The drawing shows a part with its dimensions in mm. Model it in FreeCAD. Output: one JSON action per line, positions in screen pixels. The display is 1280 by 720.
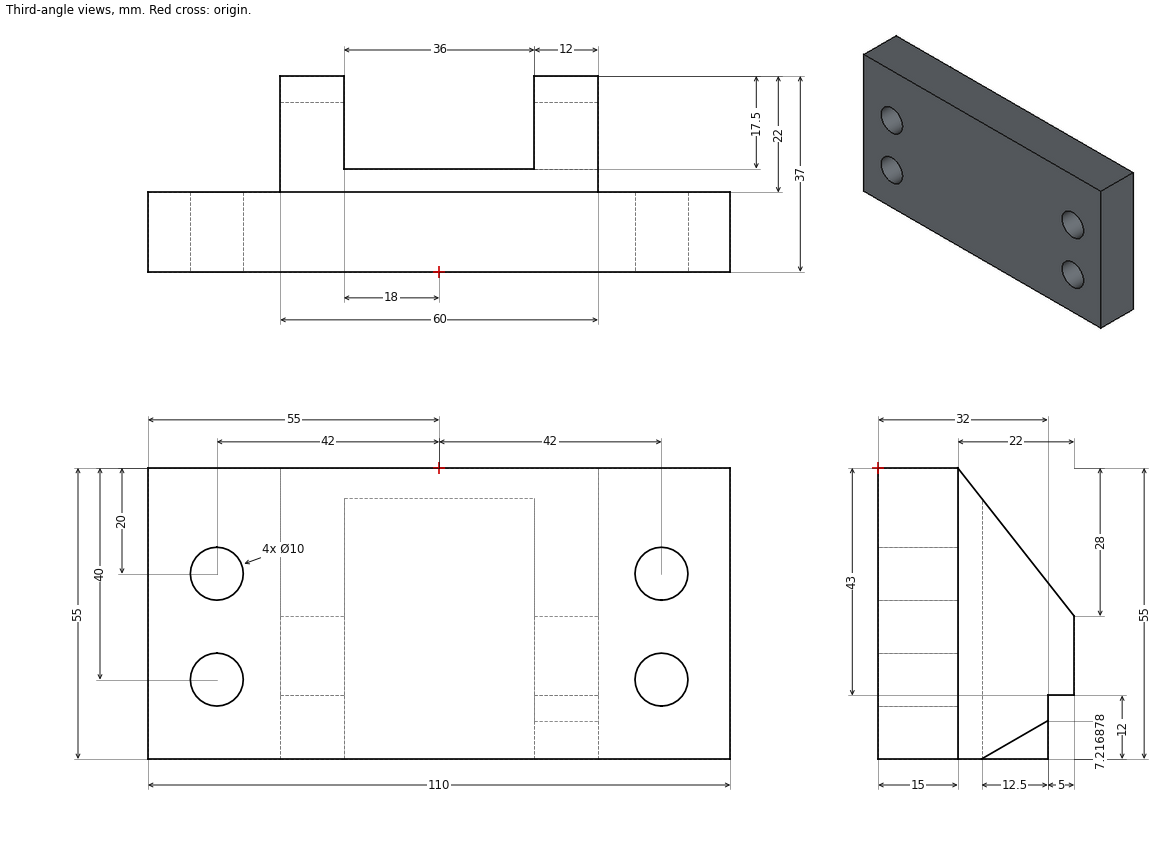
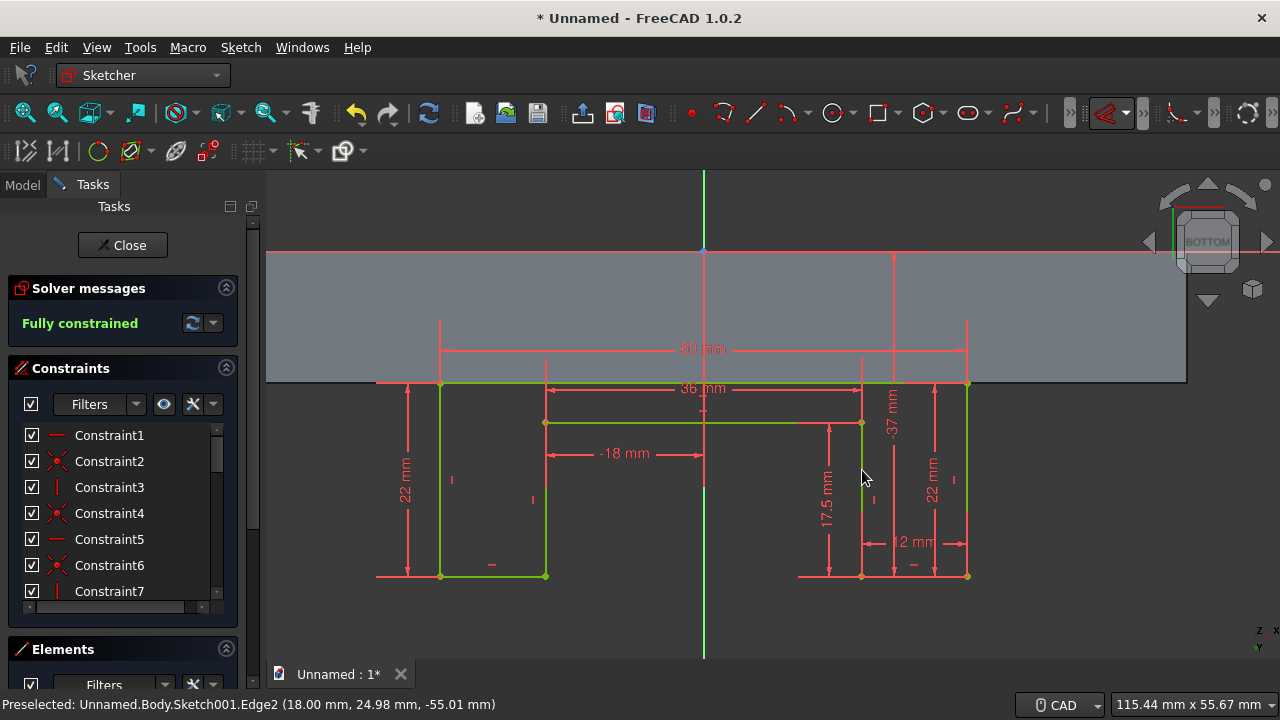
{"action": "left_click", "coordinate": [123, 245]}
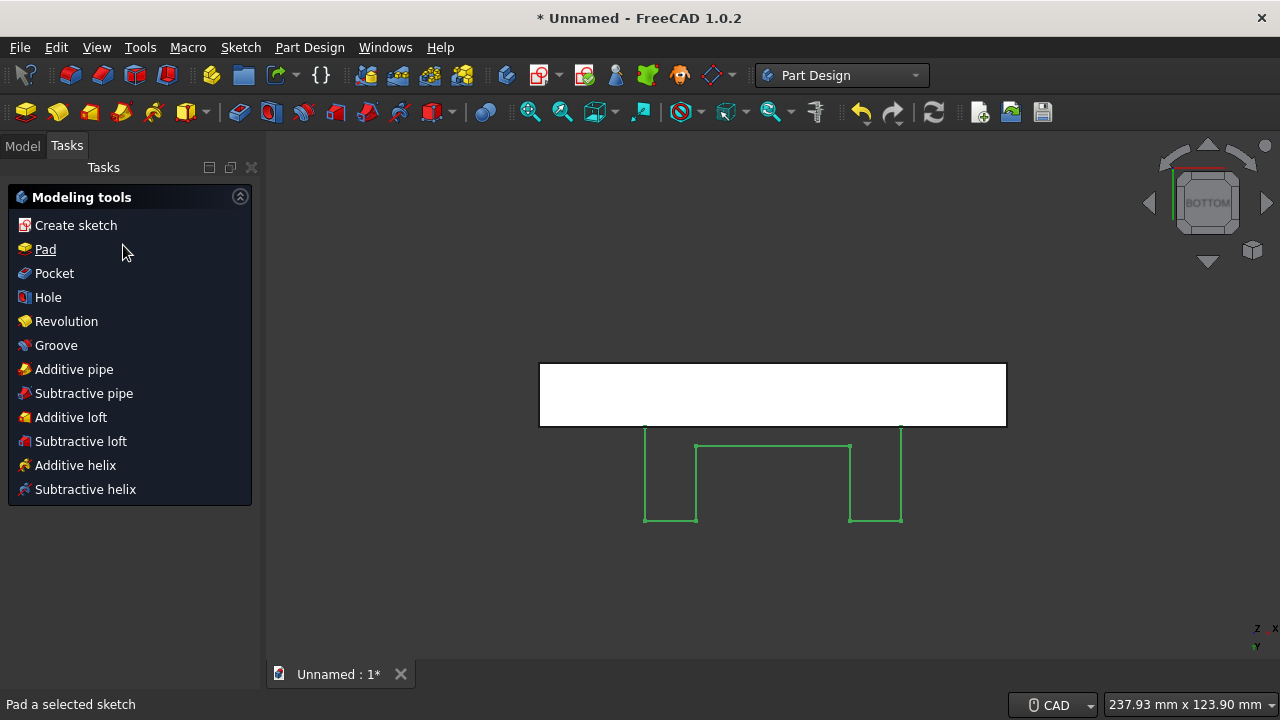
{"action": "left_click", "coordinate": [26, 112]}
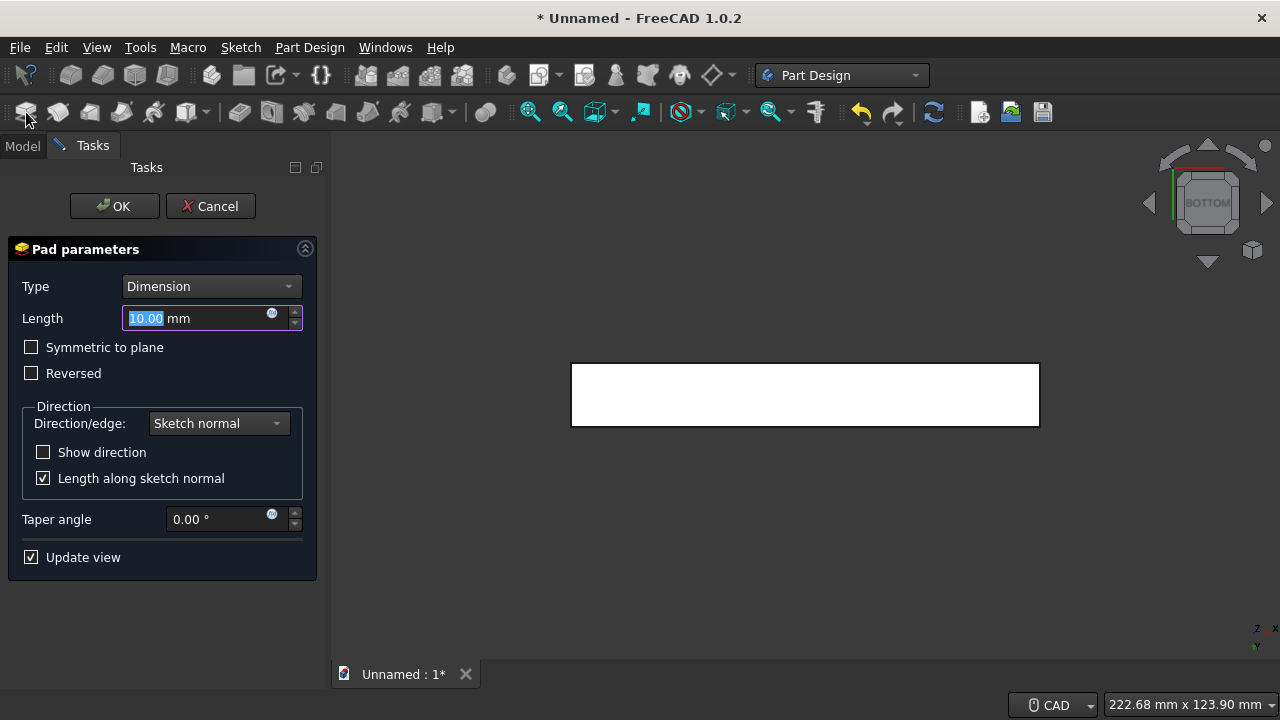
{"action": "type", "text": "55"}
{"action": "key", "text": "Tab"}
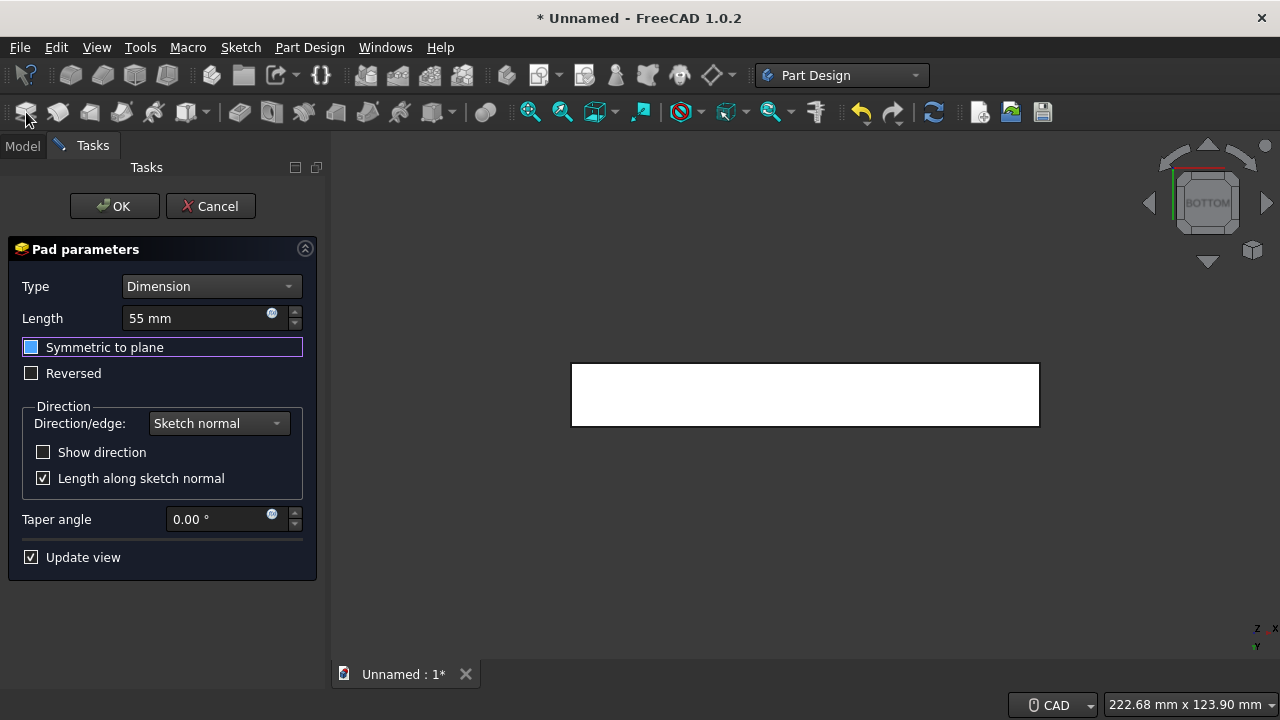
{"action": "left_click", "coordinate": [30, 373]}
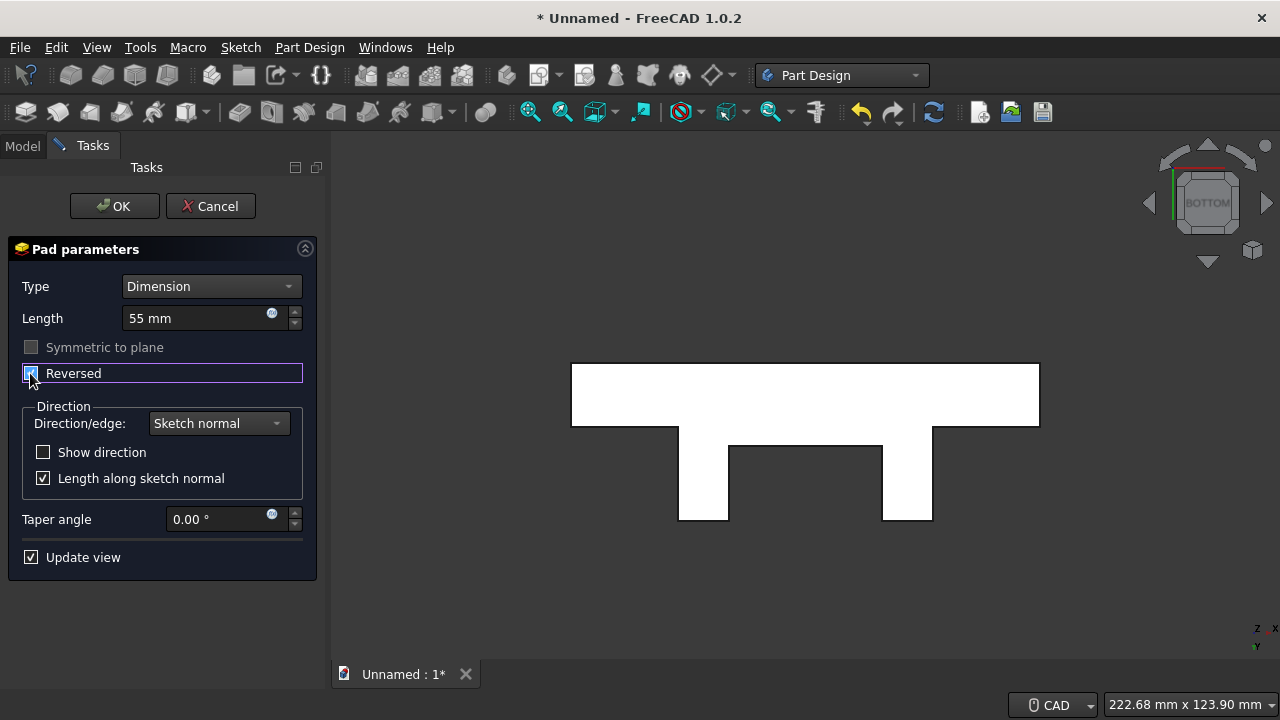
{"action": "left_click", "coordinate": [115, 206]}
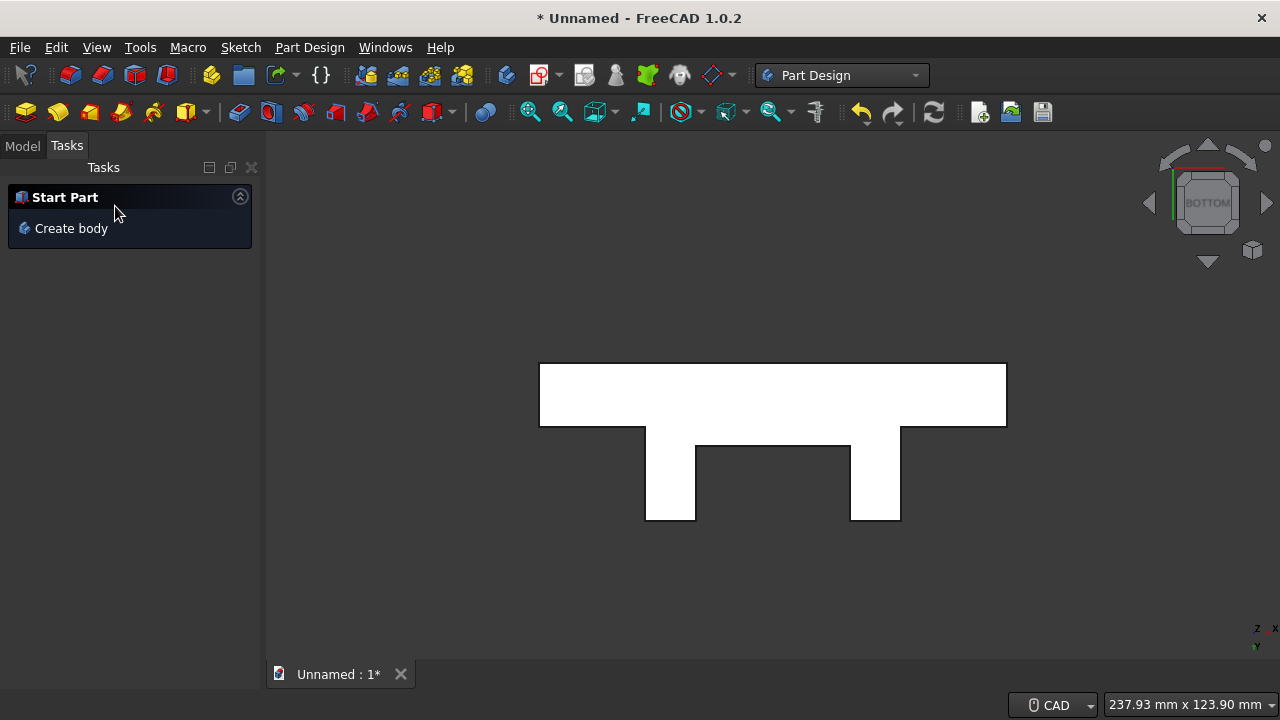
{"action": "key", "text": "6"}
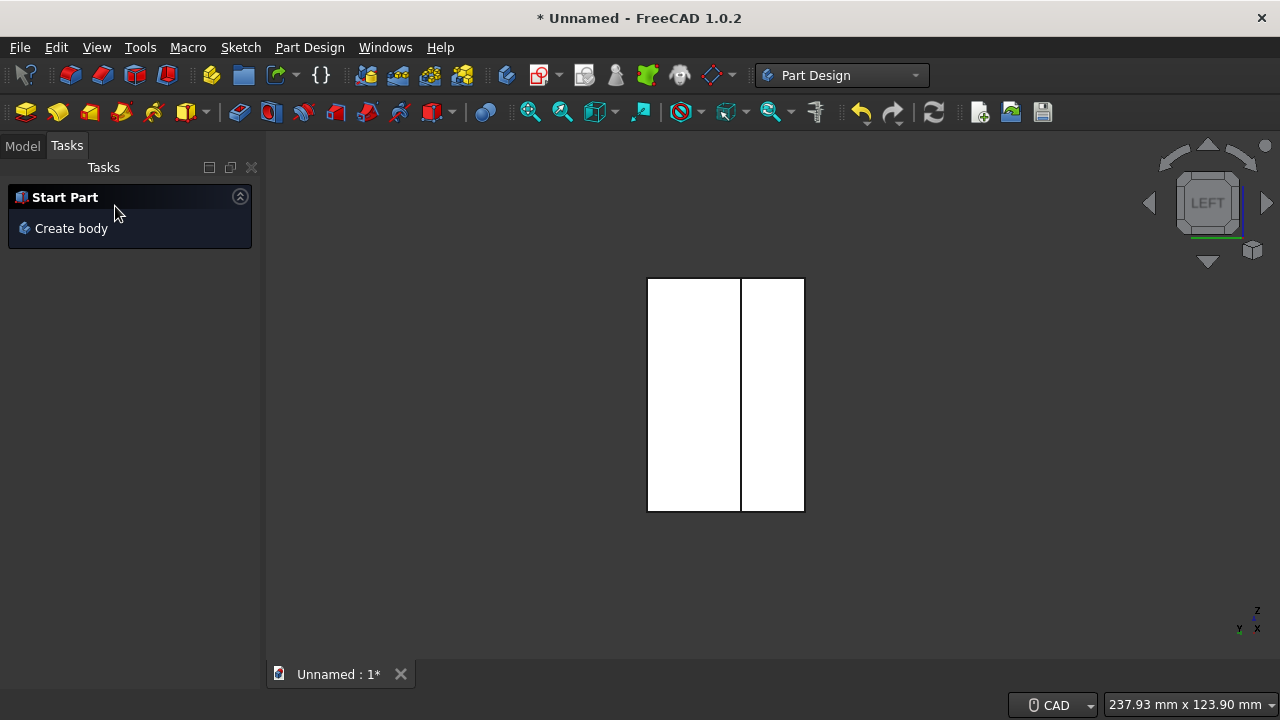
{"action": "left_click", "coordinate": [532, 112]}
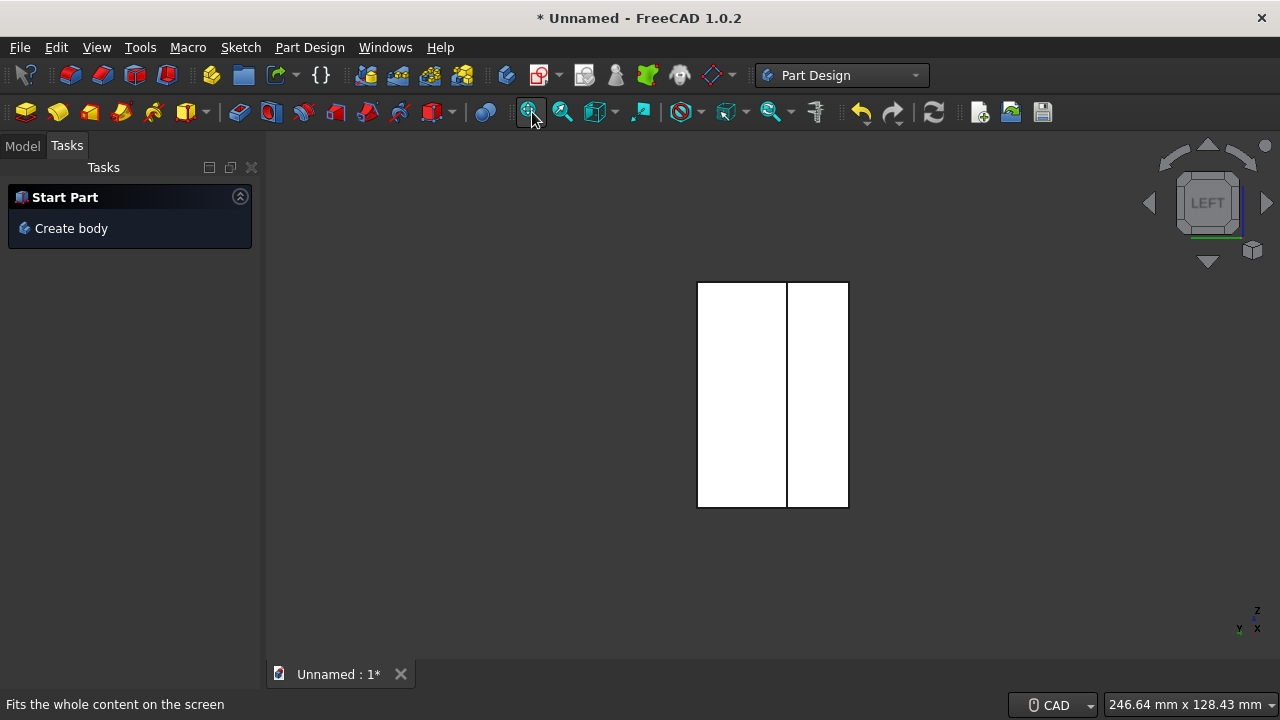
{"action": "left_click", "coordinate": [742, 329]}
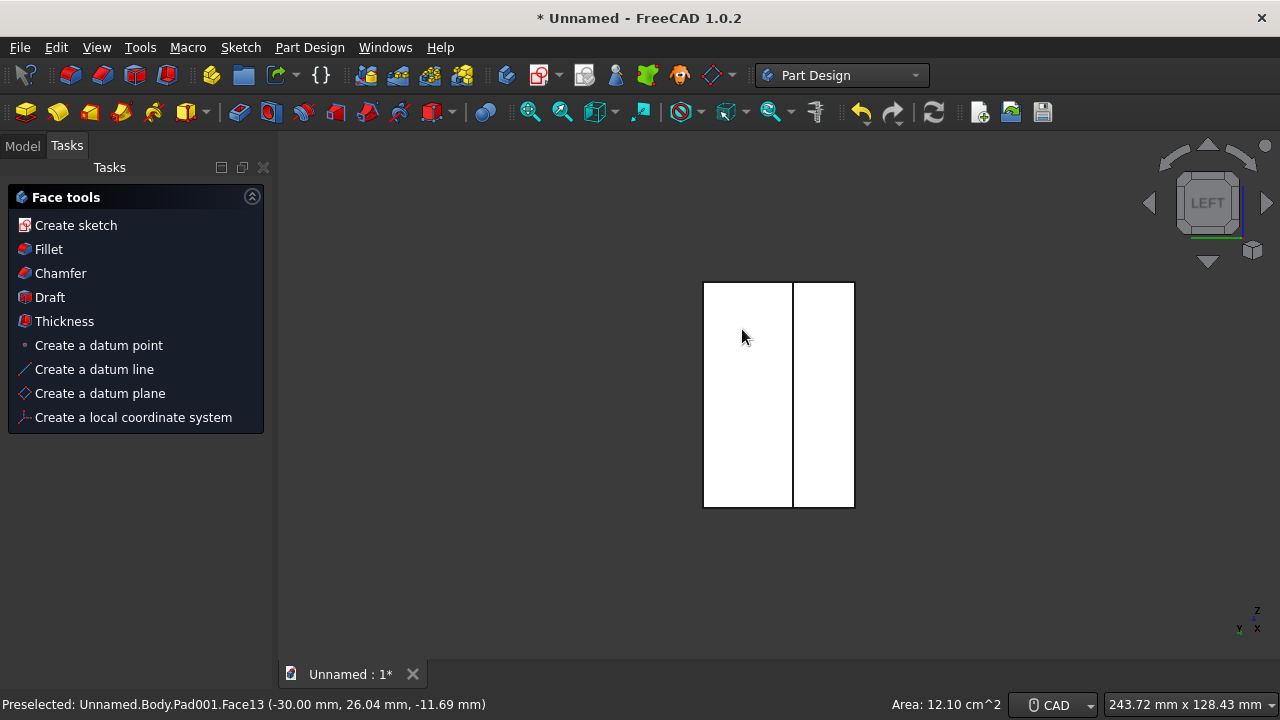
{"action": "left_click", "coordinate": [540, 76]}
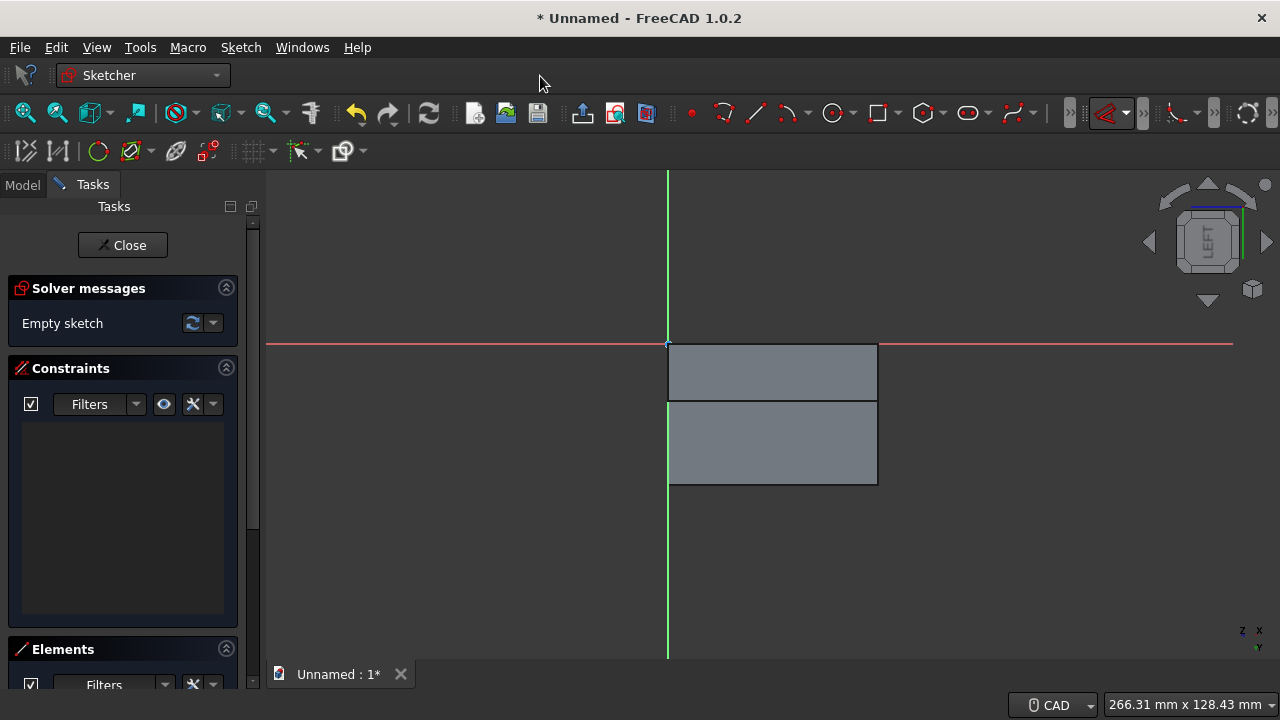
{"action": "left_click", "coordinate": [648, 114]}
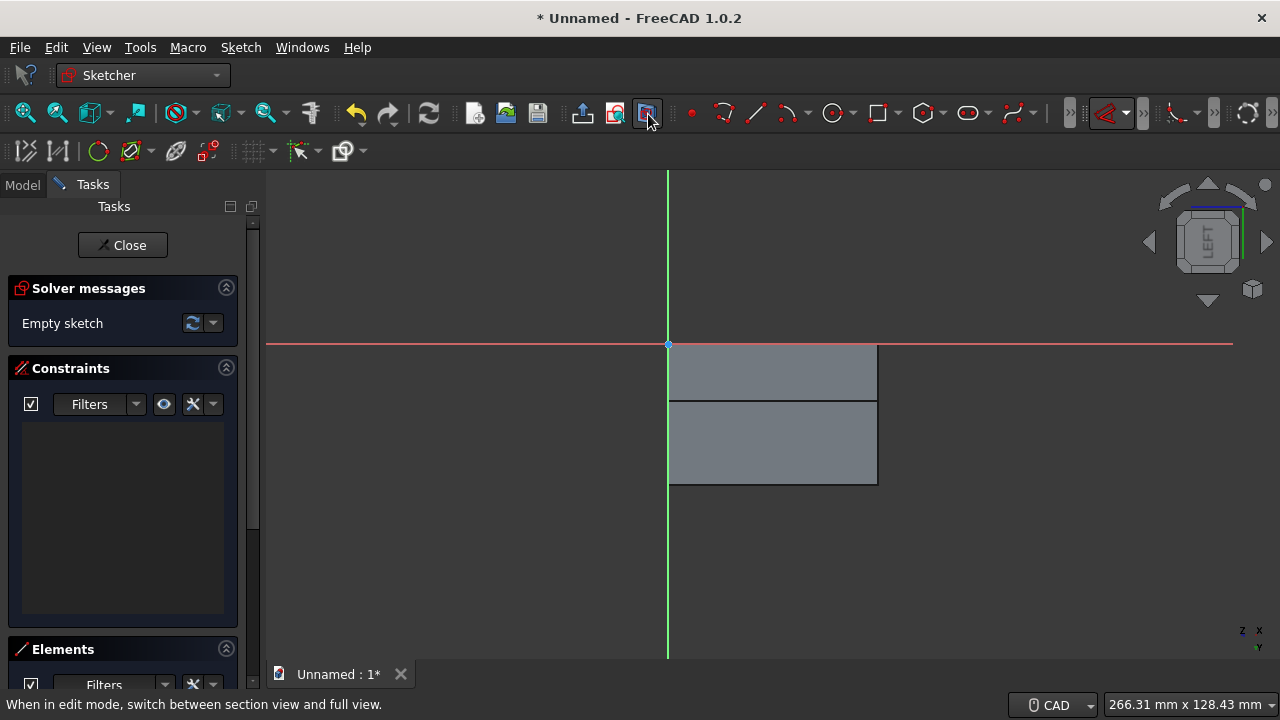
{"action": "scroll", "coordinate": [829, 414], "scroll_direction": "up", "scroll_amount": 4}